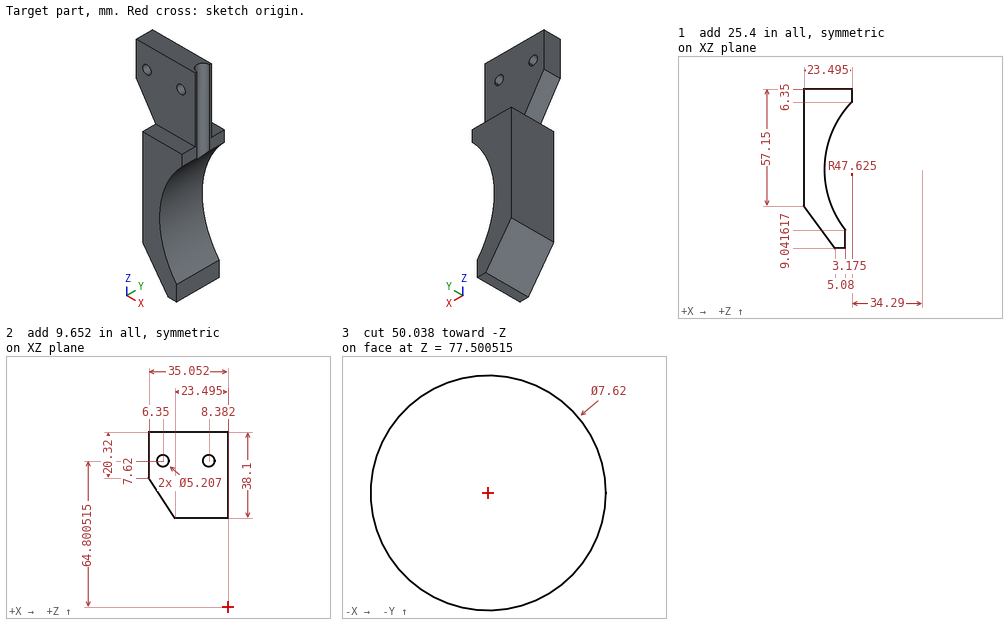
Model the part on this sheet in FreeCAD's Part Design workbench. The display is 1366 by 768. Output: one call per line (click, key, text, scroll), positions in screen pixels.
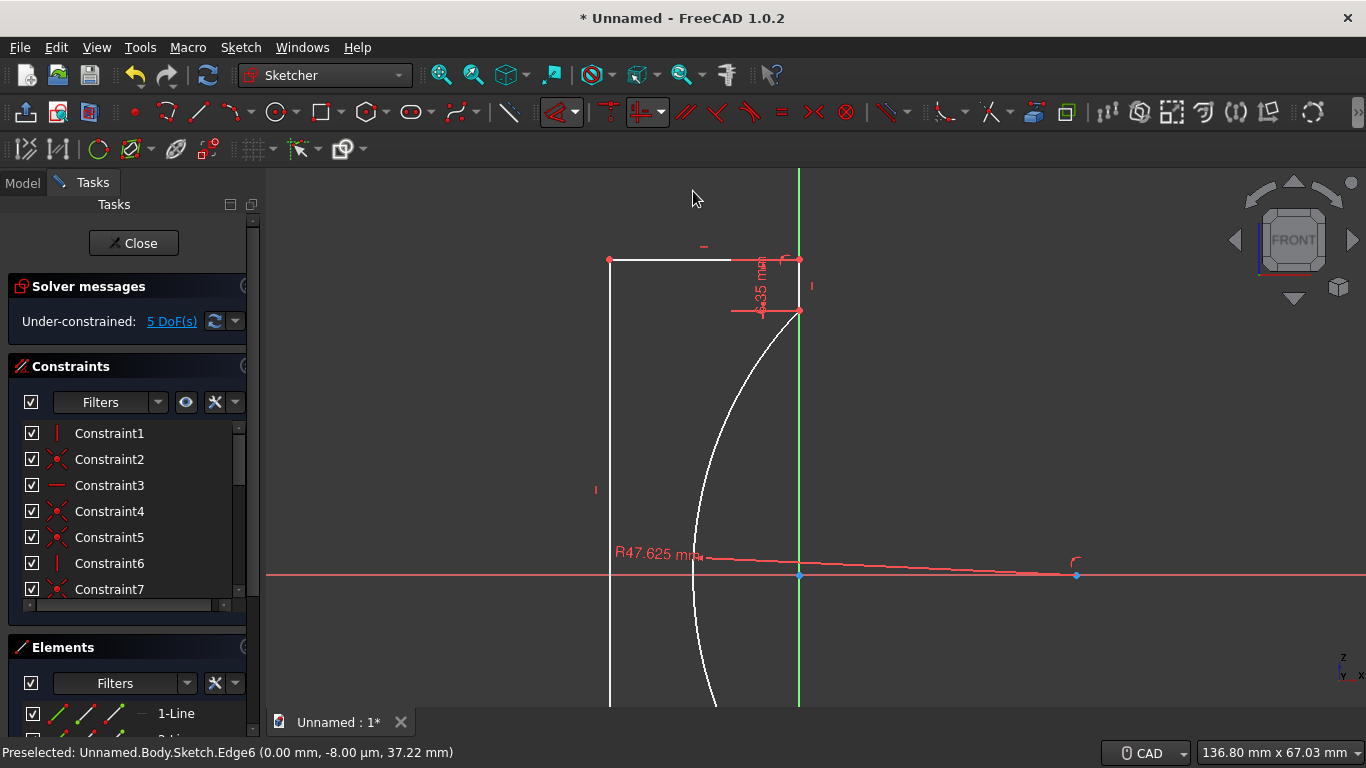
click(610, 398)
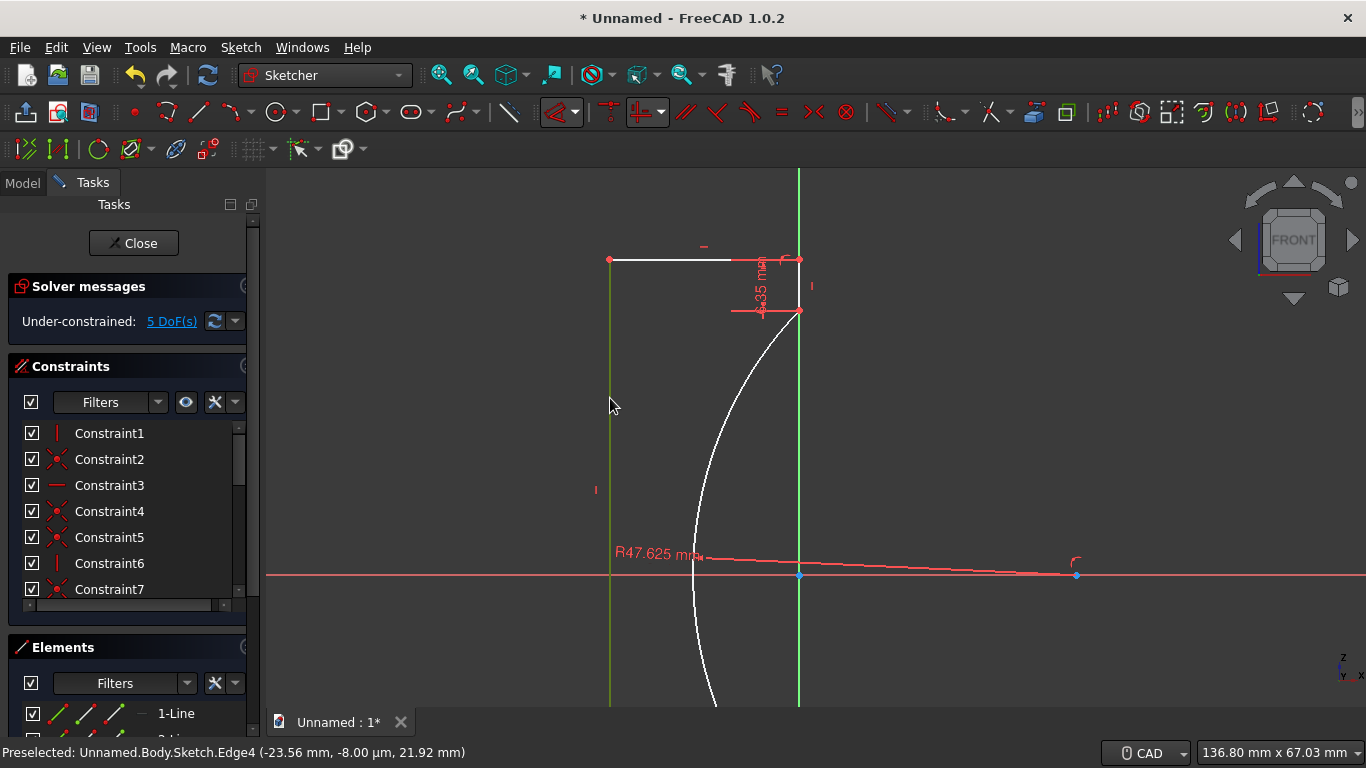
key(i)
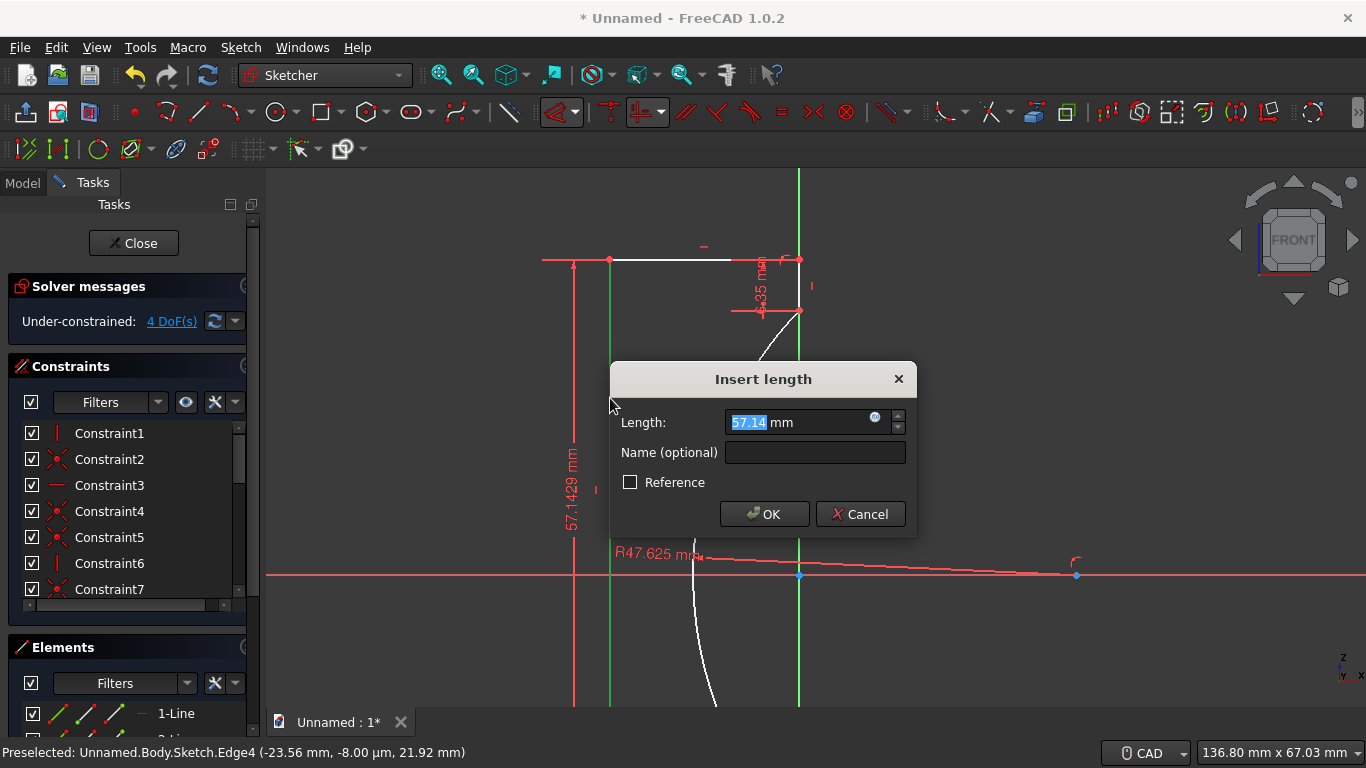
text(57.15)
key(Return)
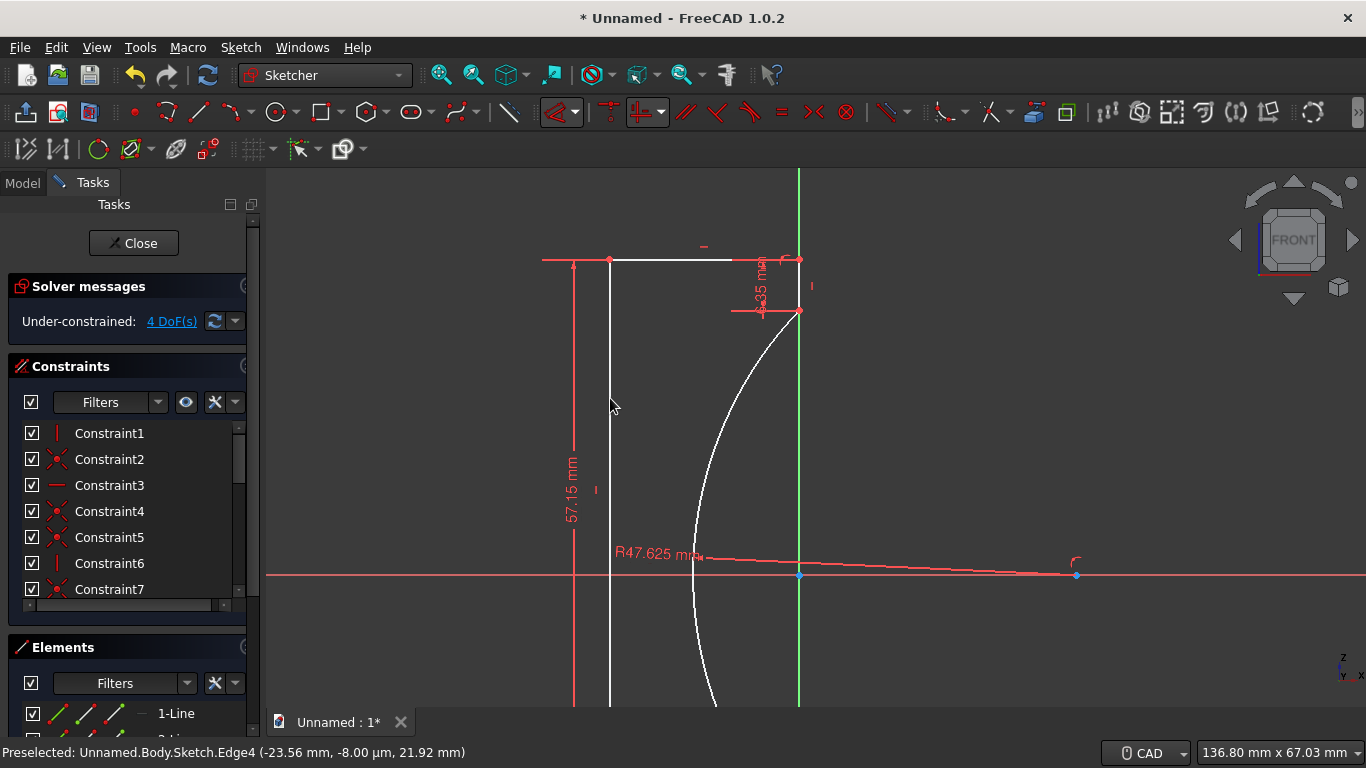
click(667, 260)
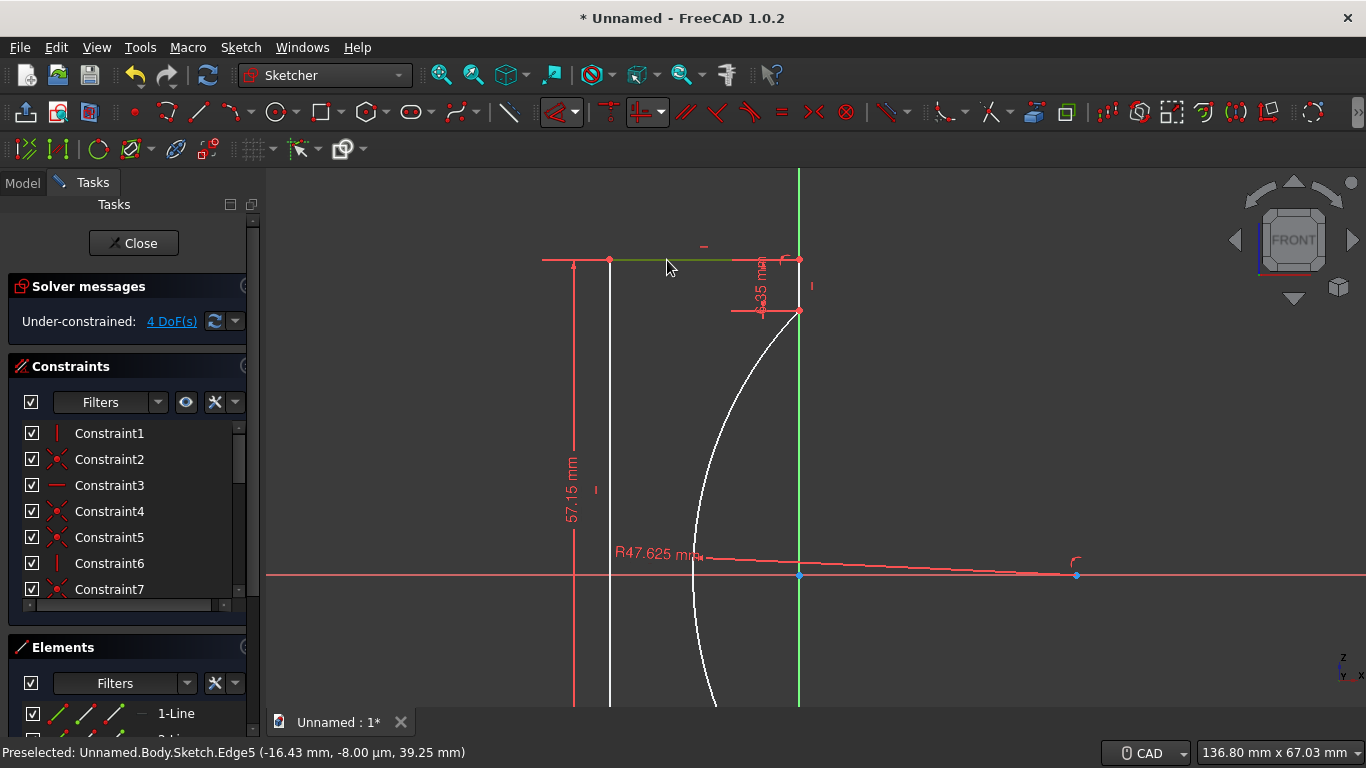
click(578, 112)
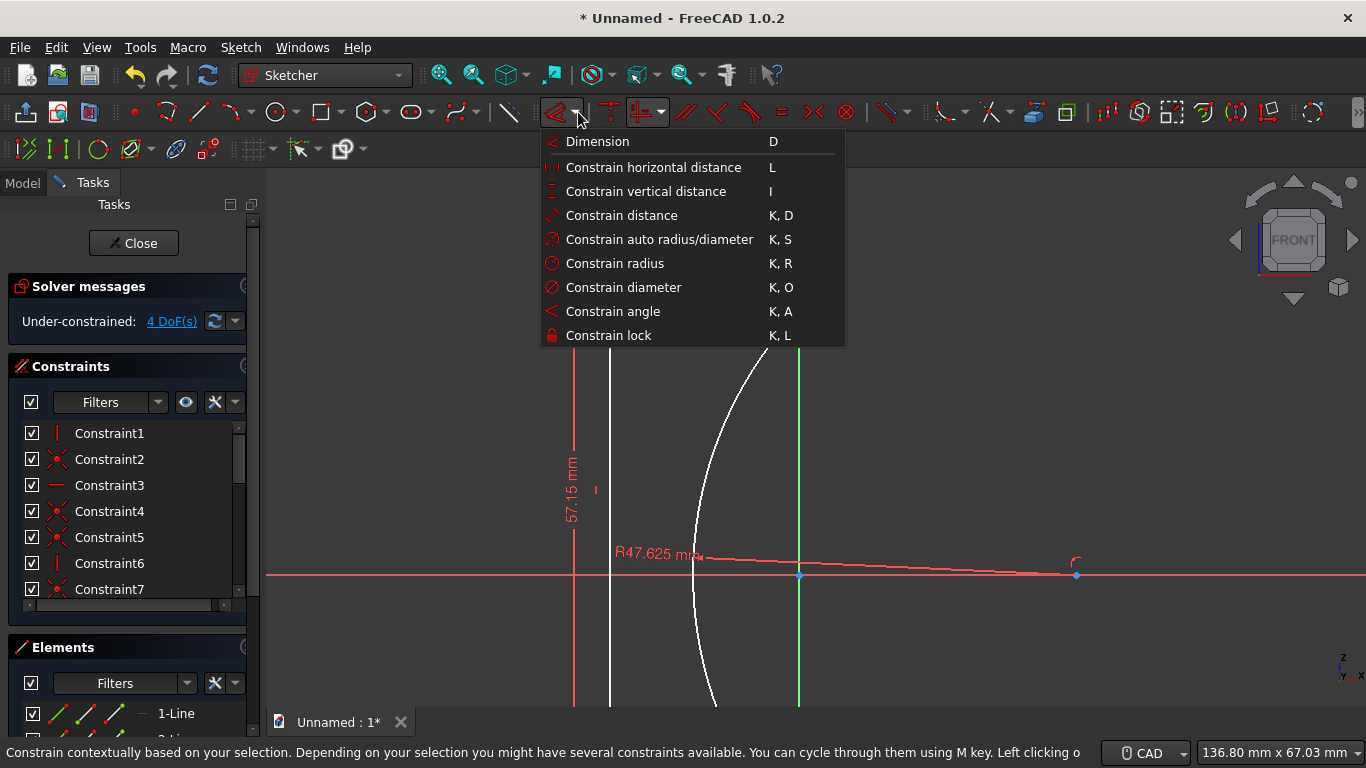
click(693, 167)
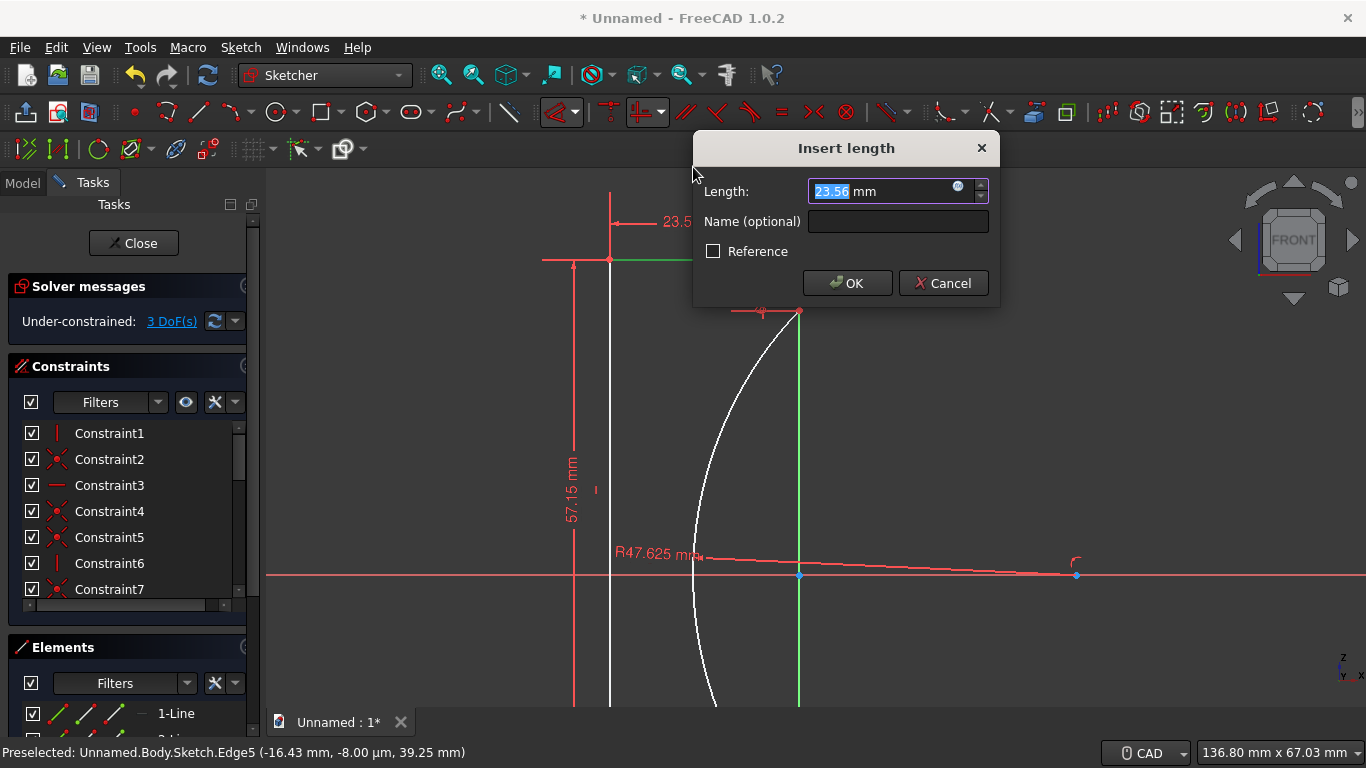
text(23.495)
key(Return)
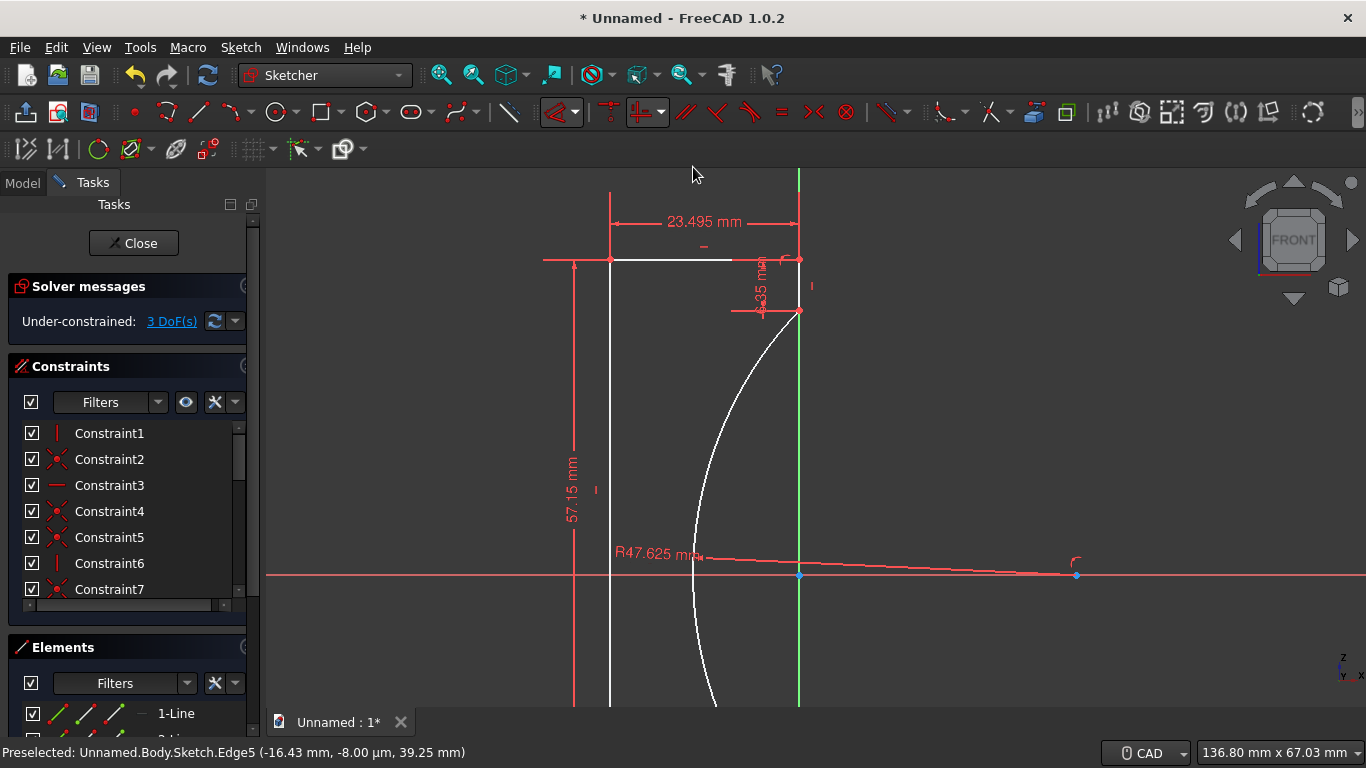
scroll(800, 275, down, 3)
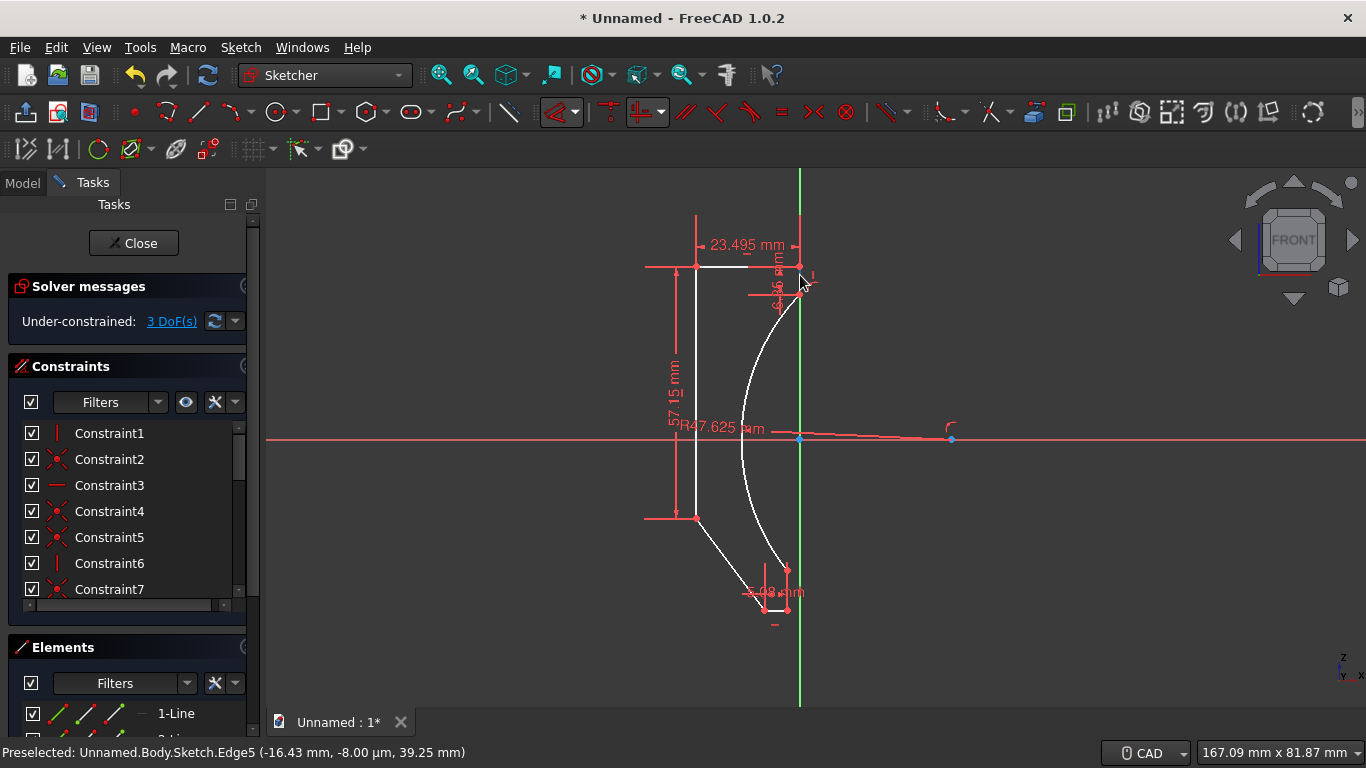
scroll(787, 570, up, 6)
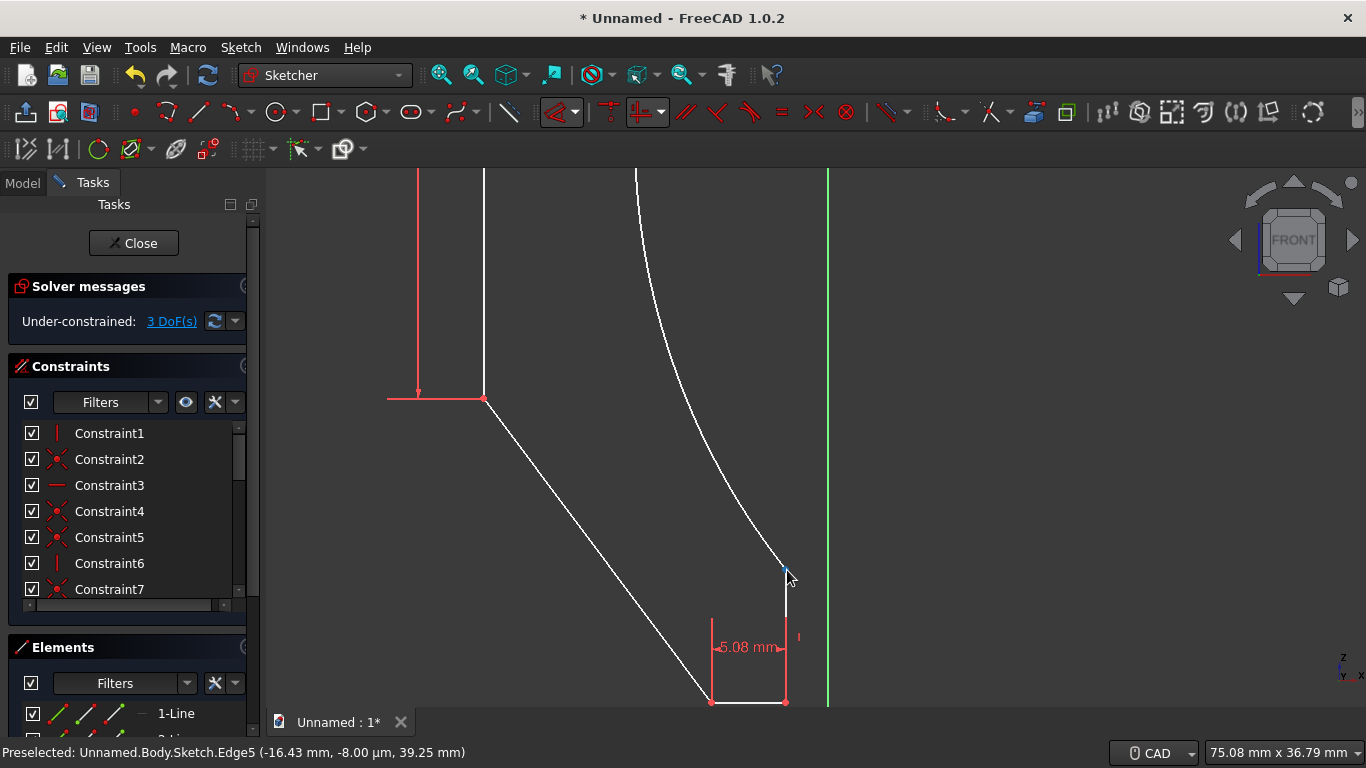
click(786, 570)